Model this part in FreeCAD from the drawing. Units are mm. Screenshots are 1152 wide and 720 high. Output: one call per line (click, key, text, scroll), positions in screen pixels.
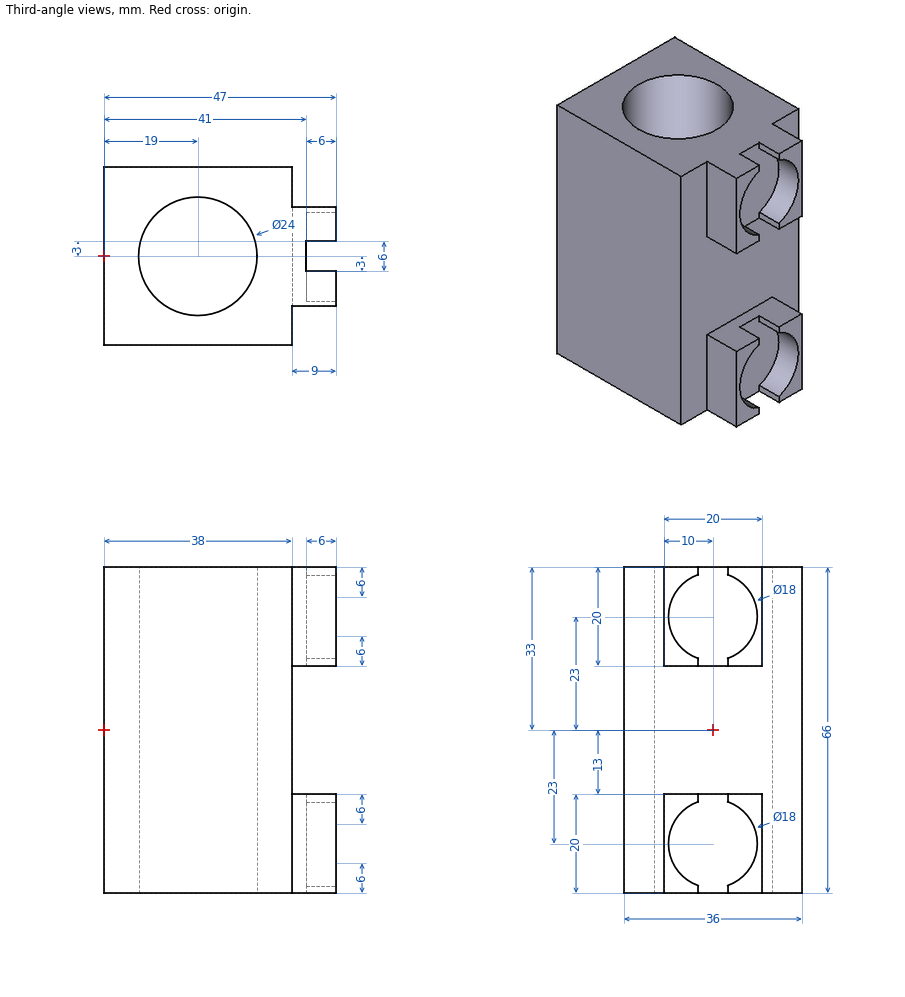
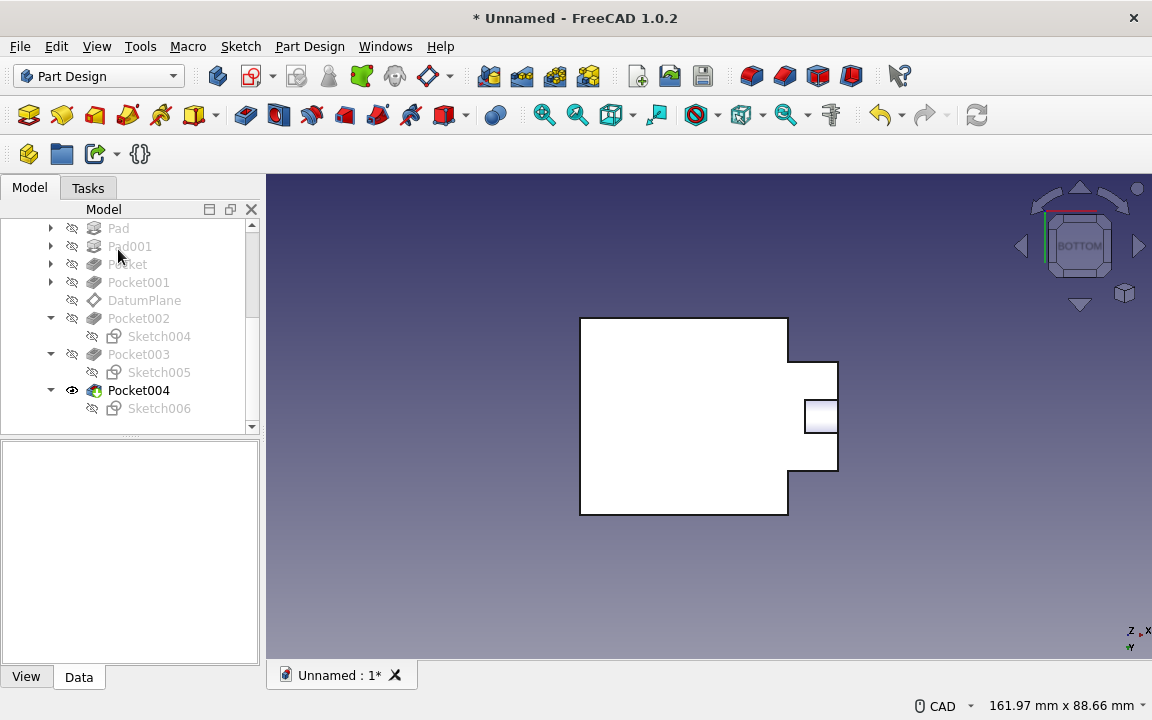
click(545, 116)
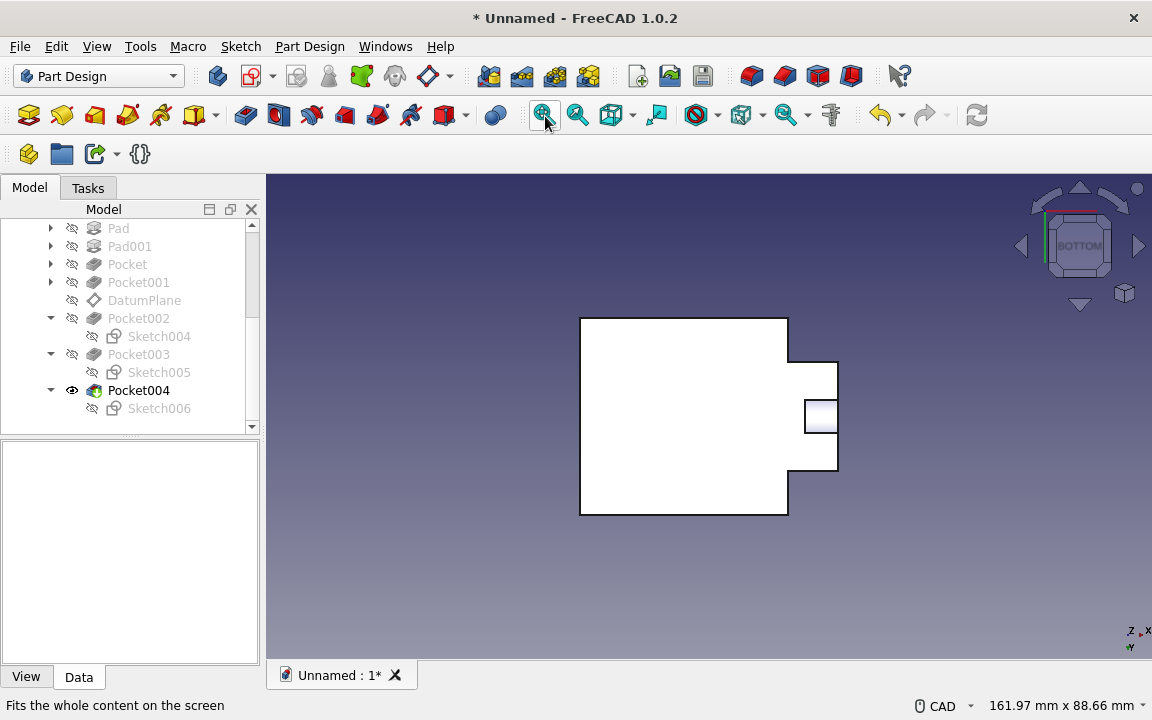
key(0)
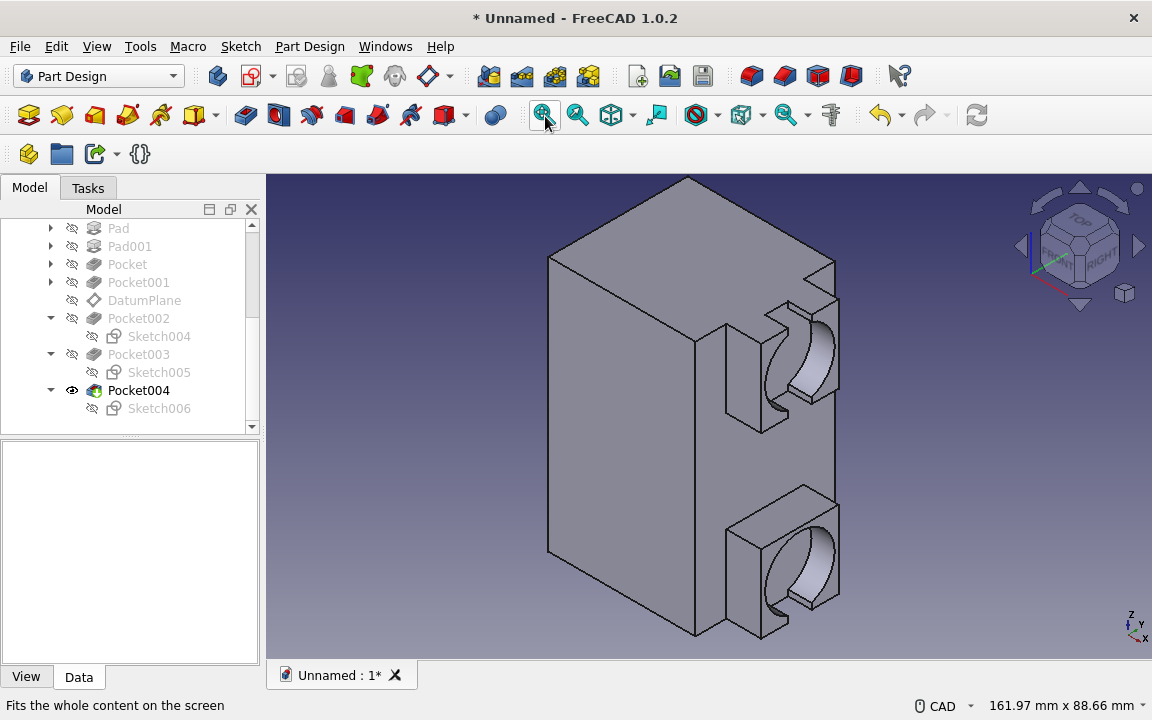
click(794, 510)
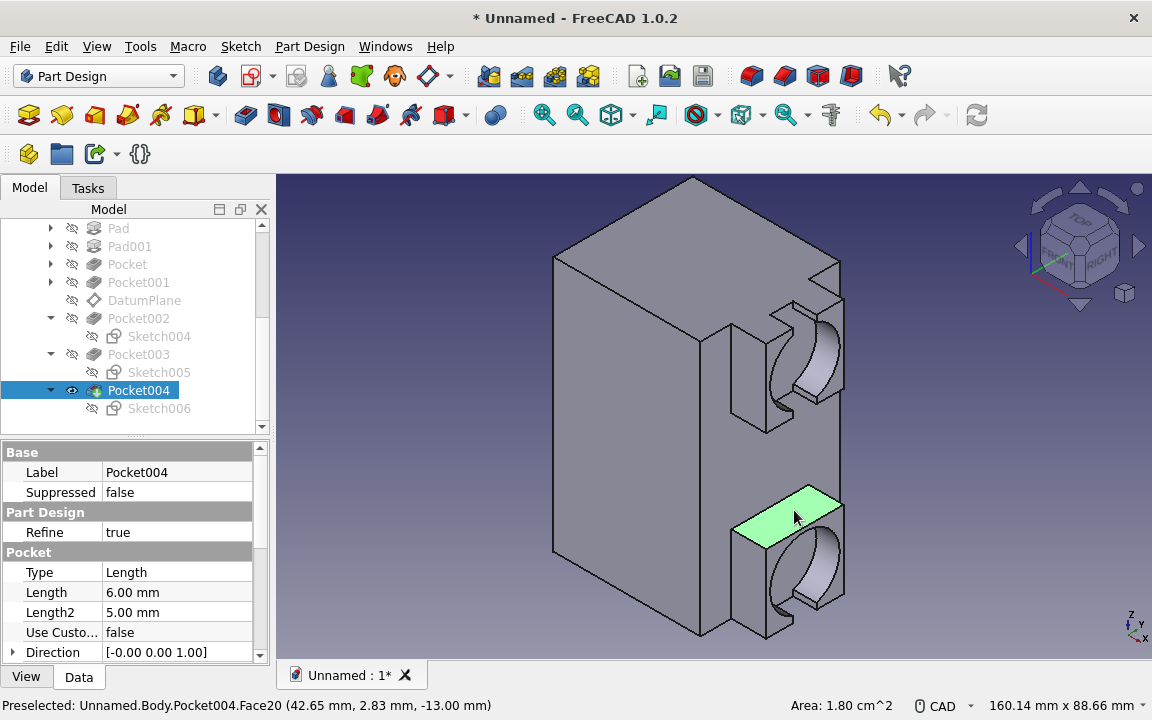
click(250, 76)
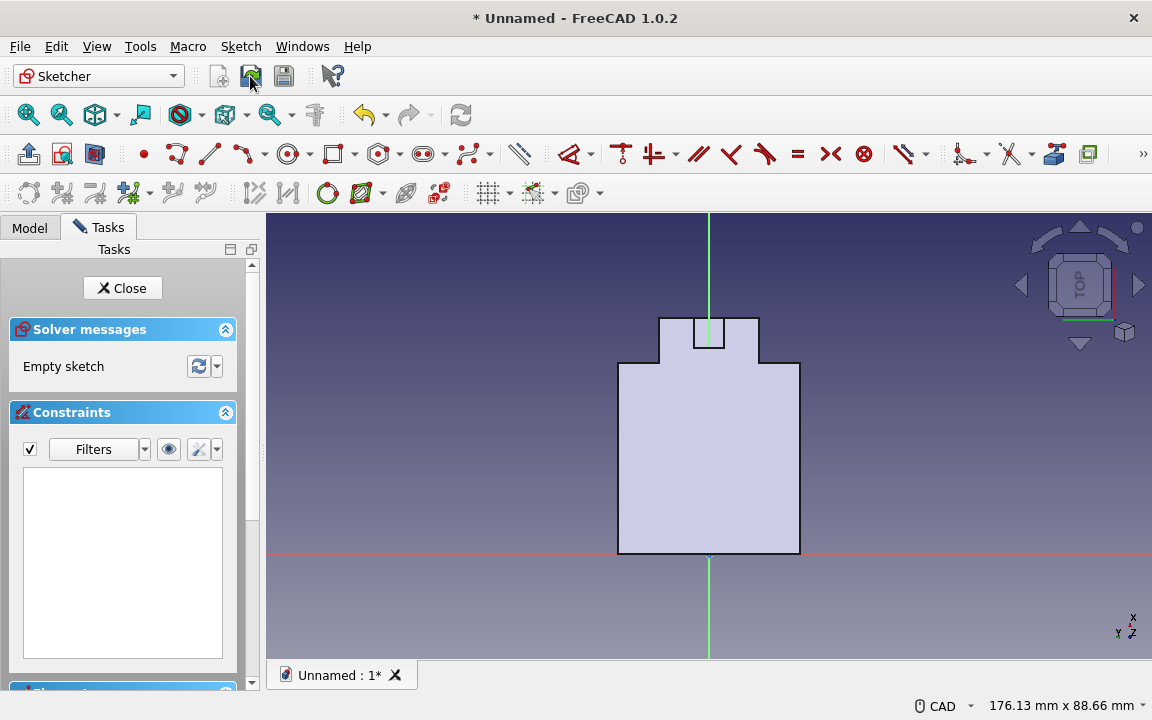
scroll(718, 320, up, 11)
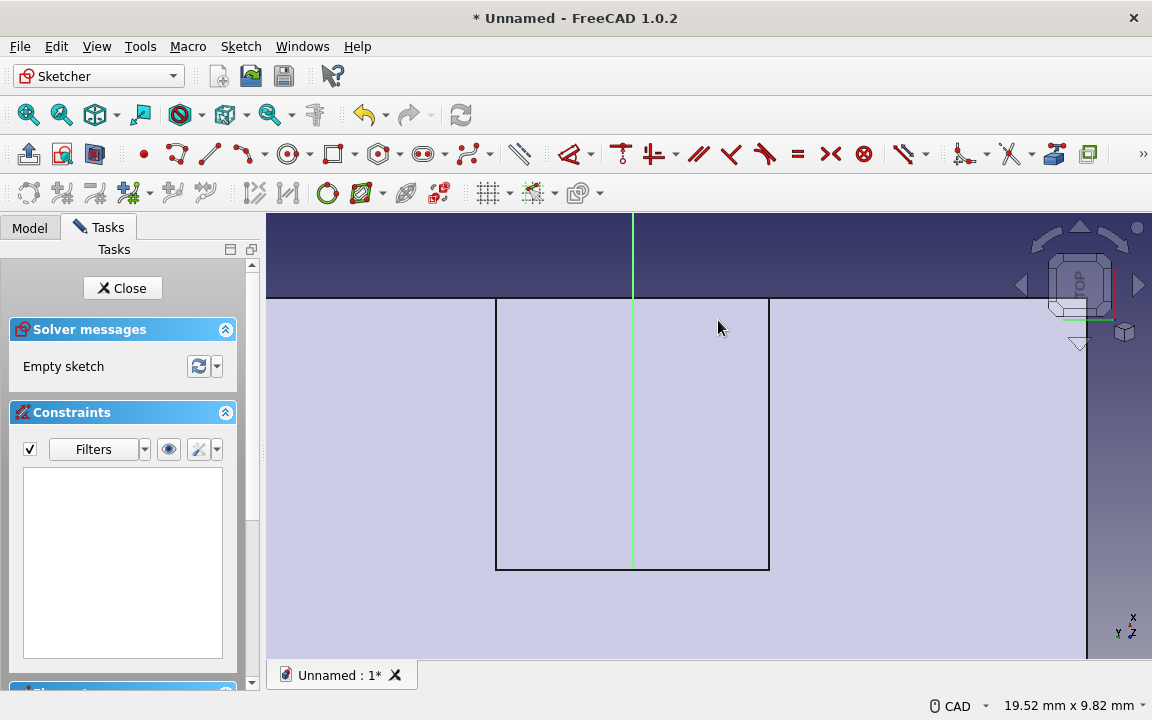
click(332, 154)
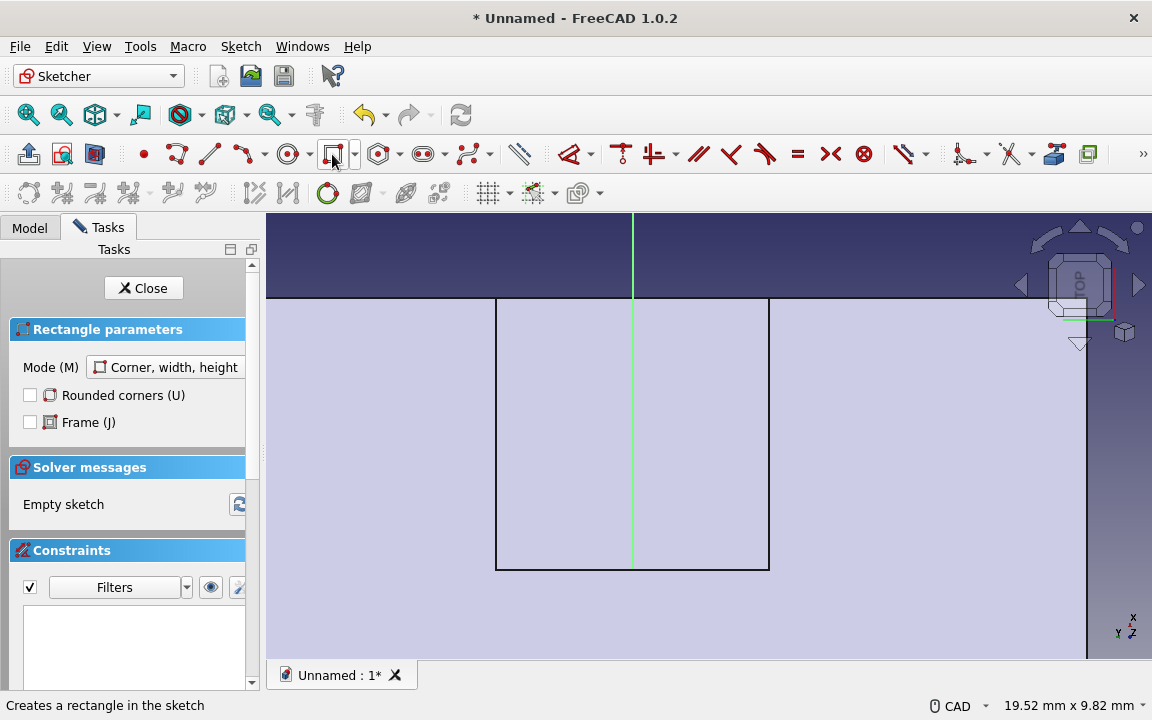
click(496, 298)
click(769, 570)
key(Escape)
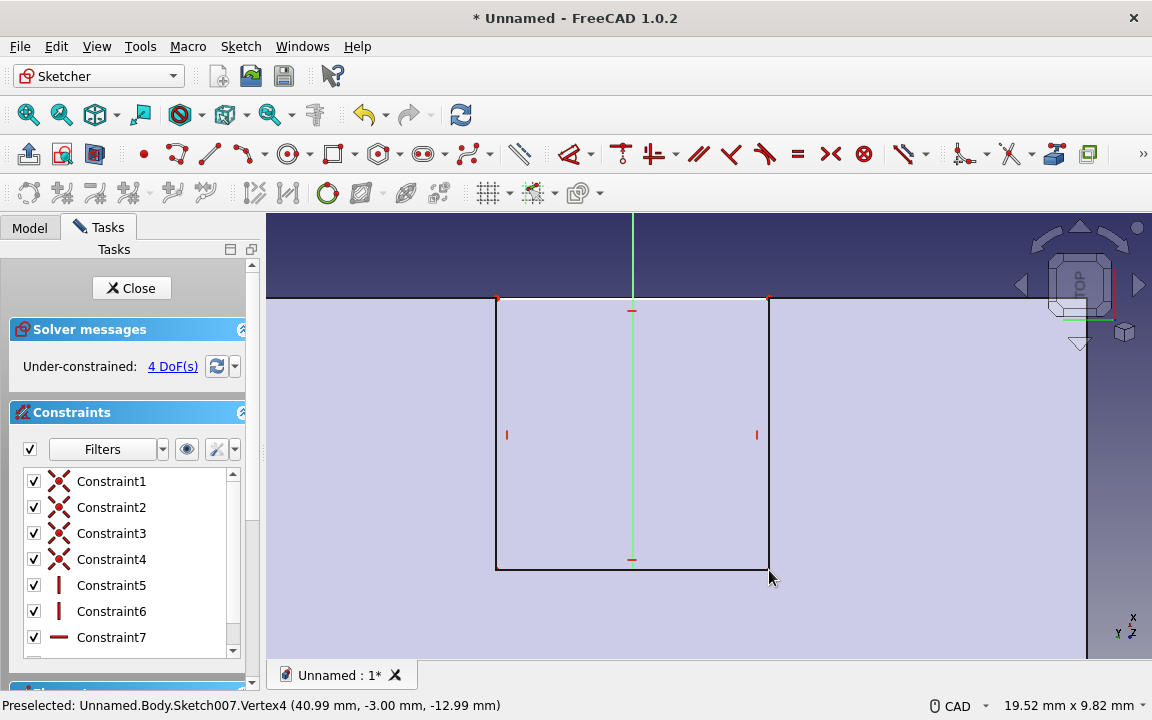
click(568, 154)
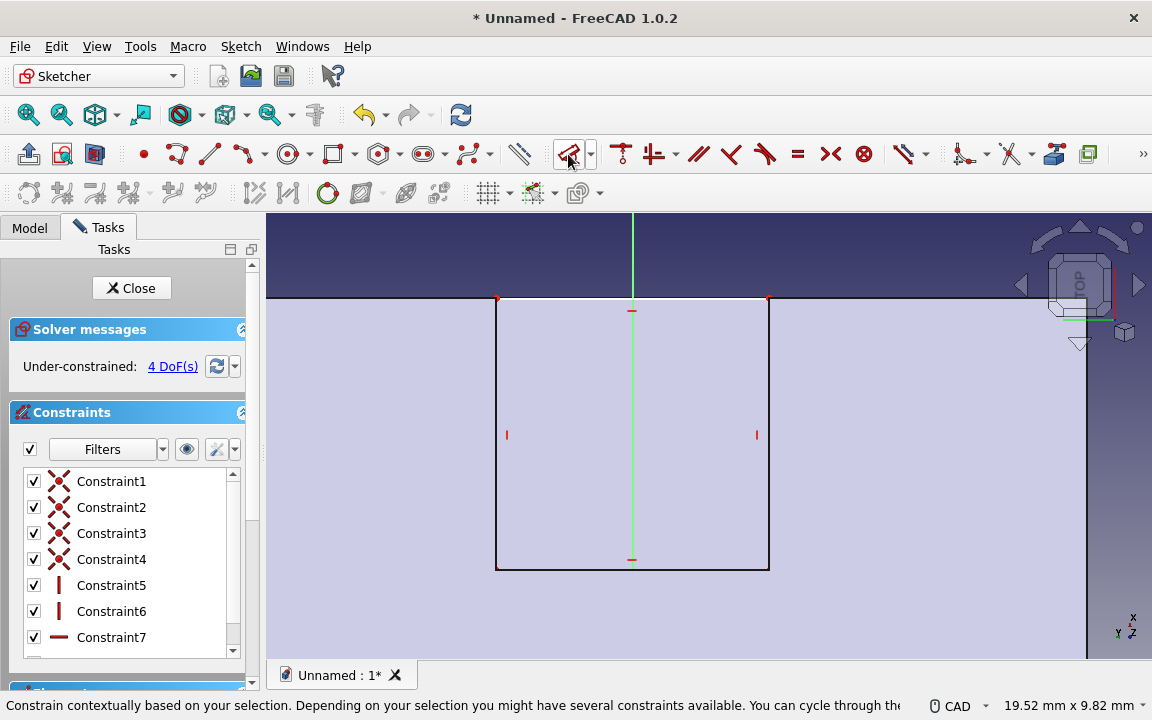
click(496, 381)
click(462, 435)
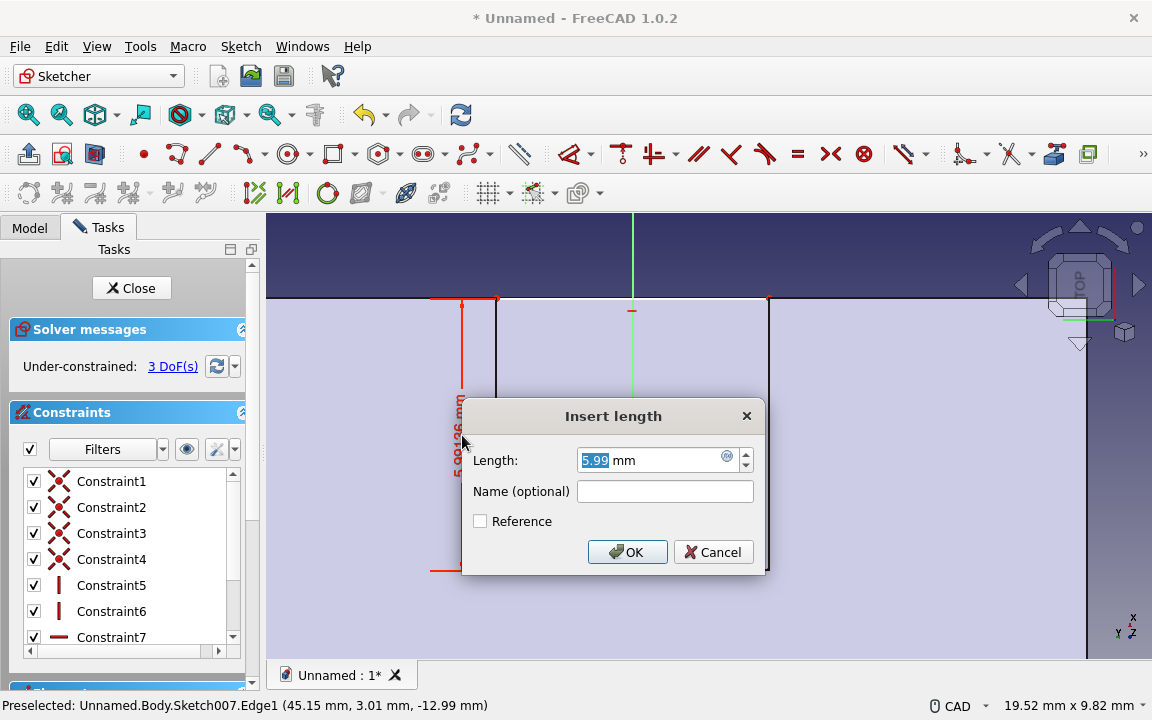
text(6)
key(Return)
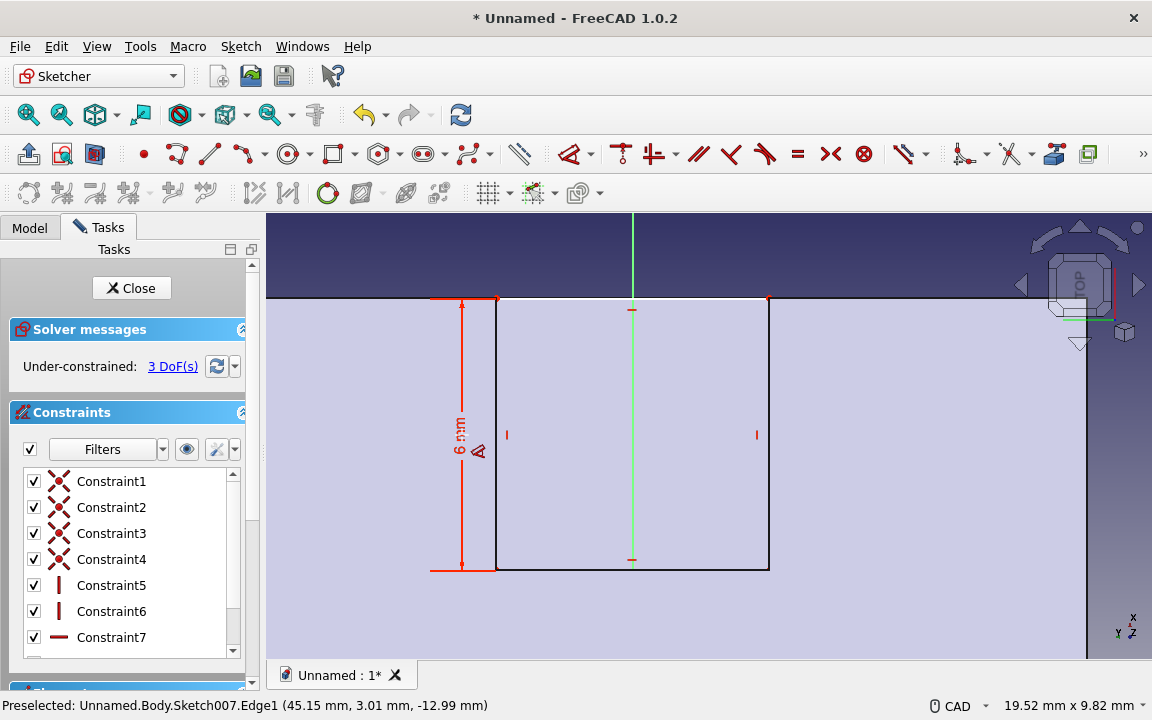
click(578, 571)
click(570, 605)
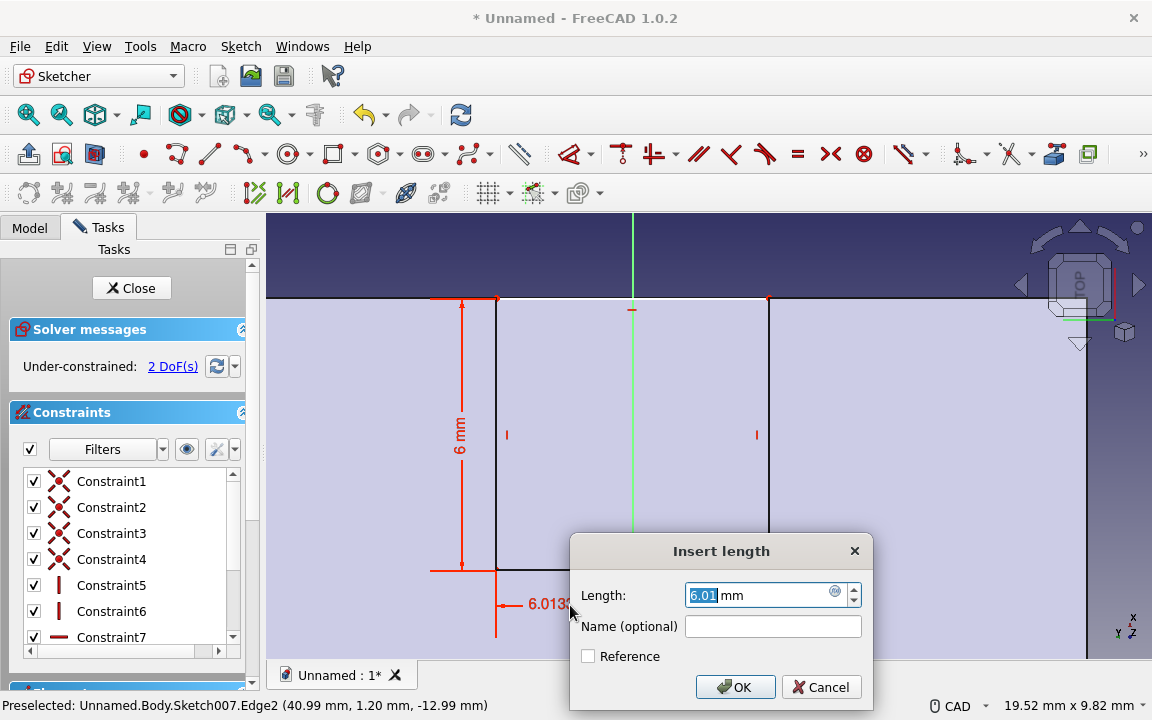
text(6)
key(Return)